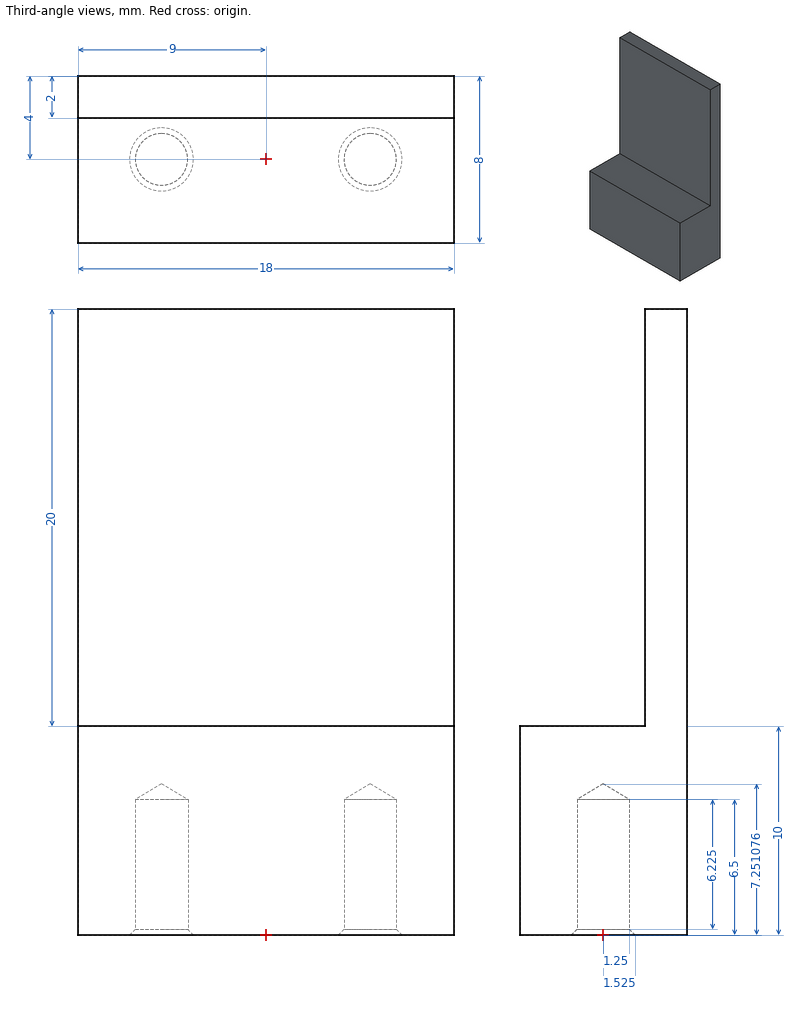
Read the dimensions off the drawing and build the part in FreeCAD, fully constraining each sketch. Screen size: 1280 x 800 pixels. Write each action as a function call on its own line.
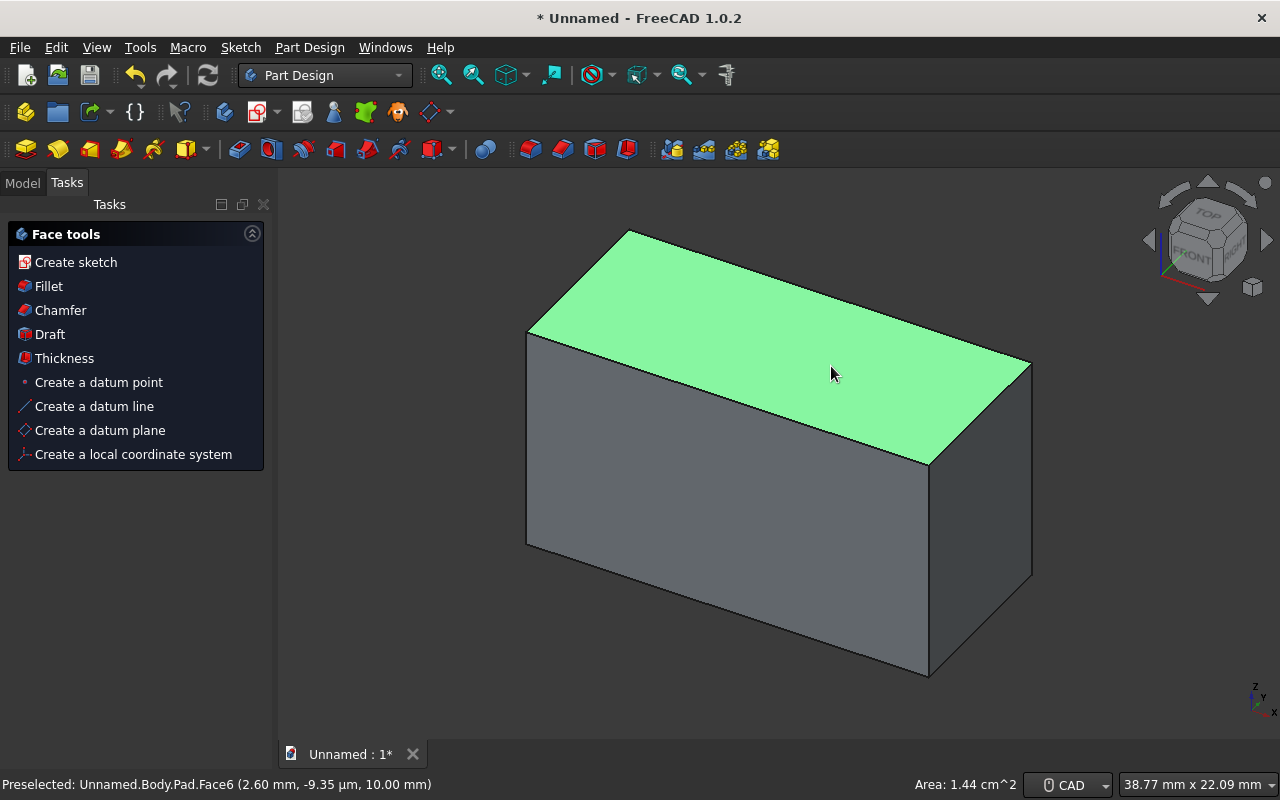
click(258, 112)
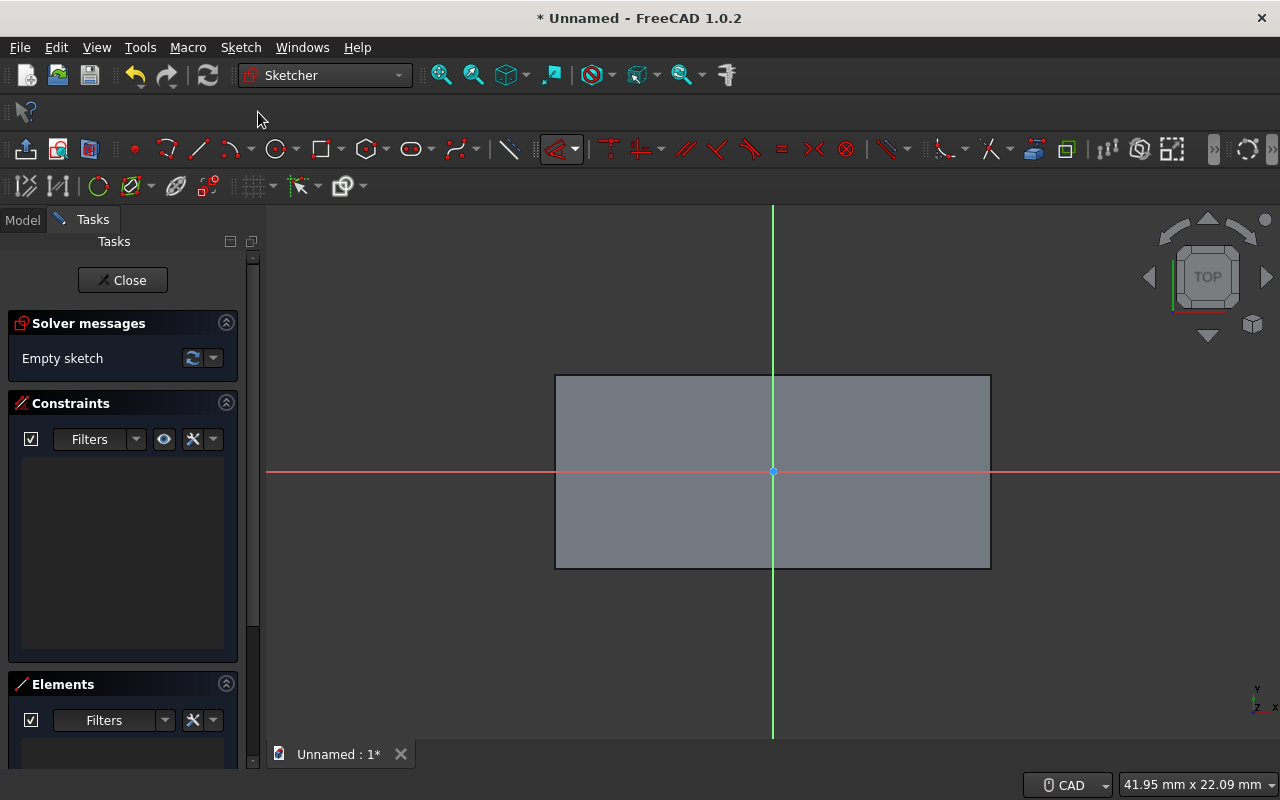
key(g)
key(r)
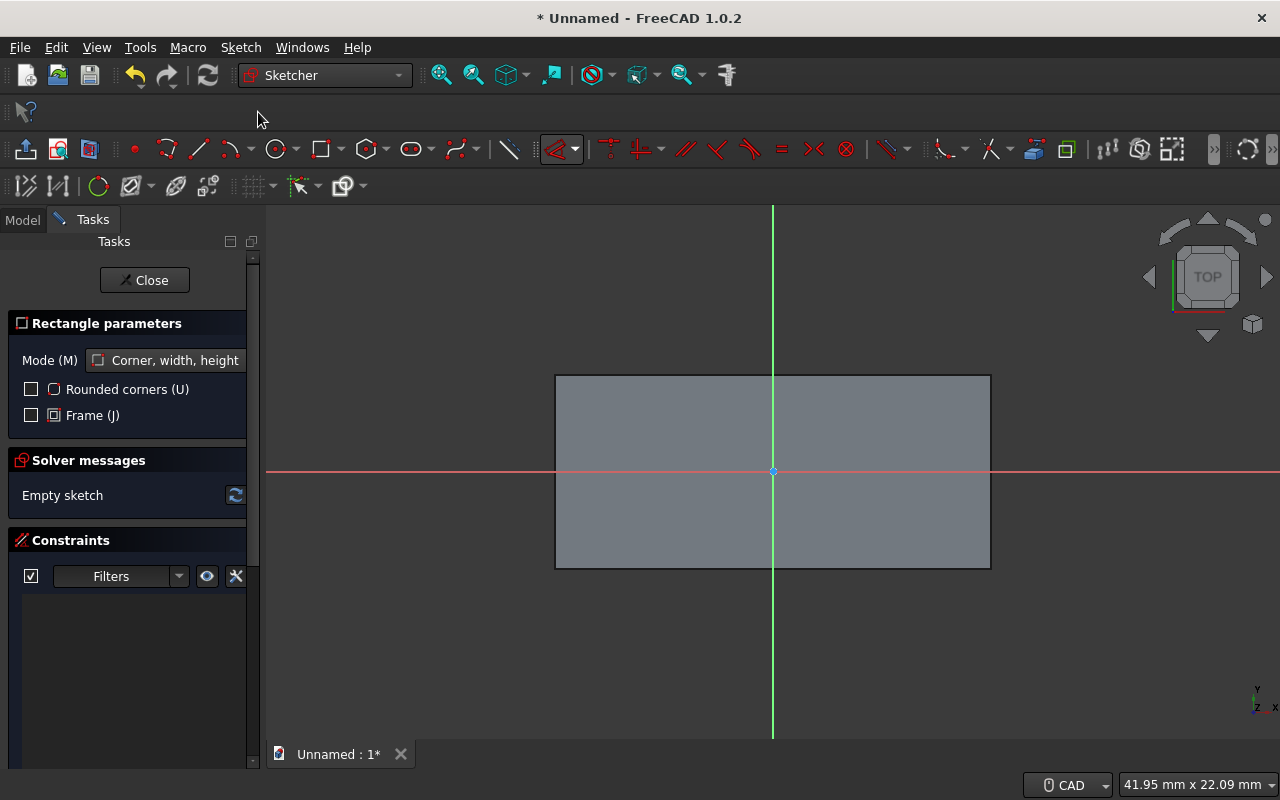
click(555, 375)
click(991, 424)
key(Escape)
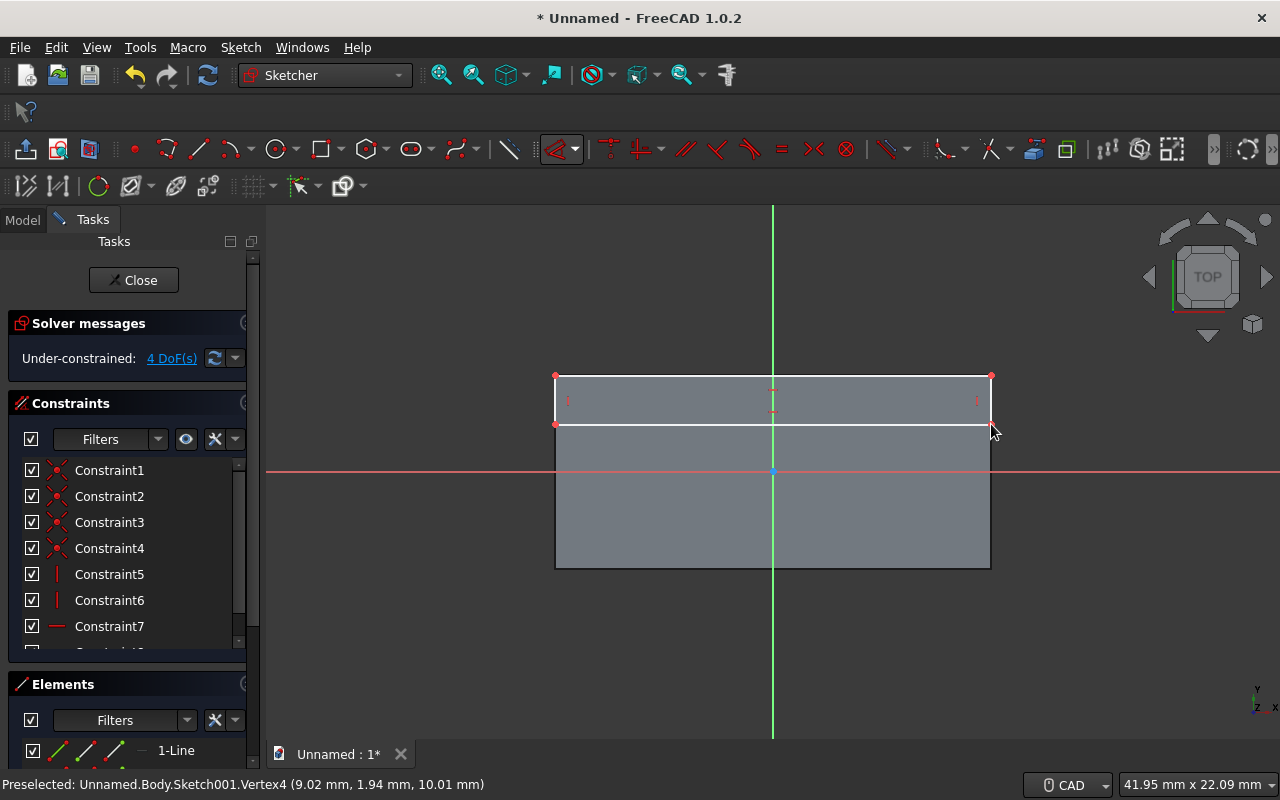
click(555, 391)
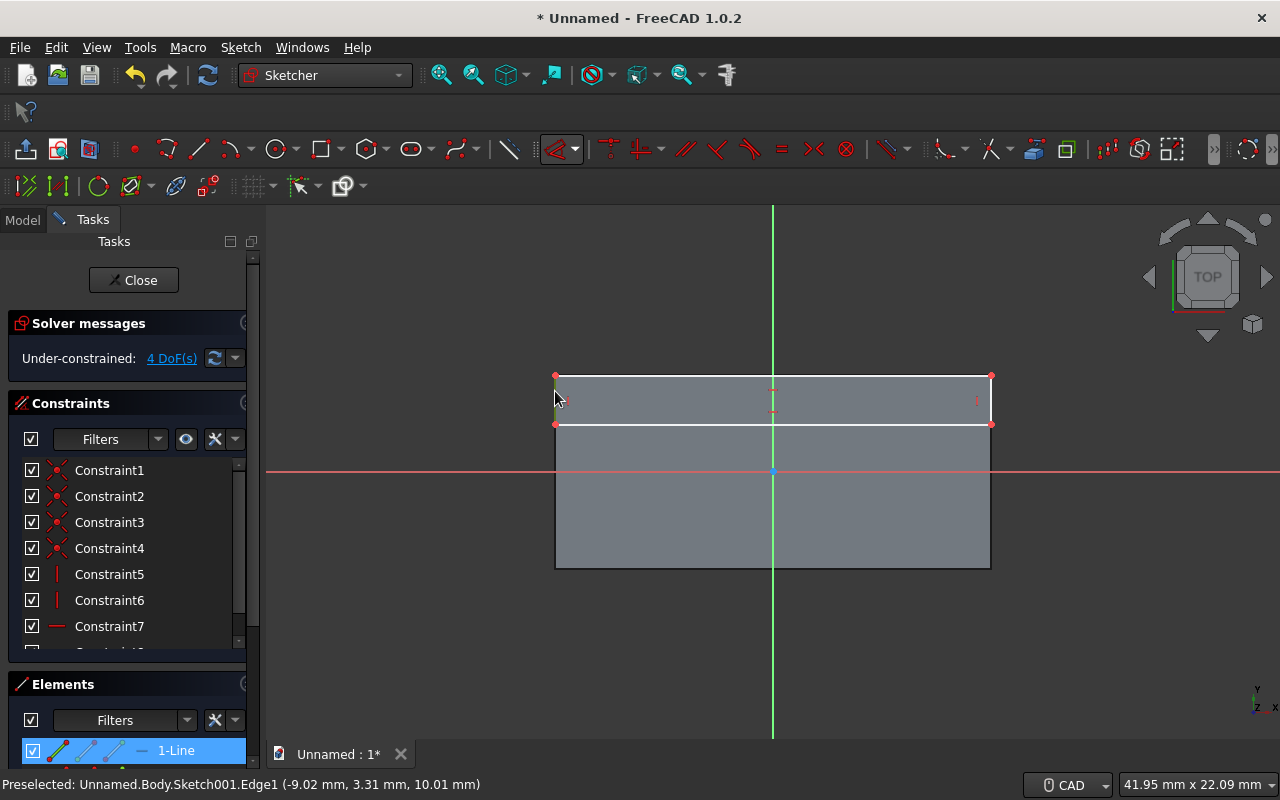
click(578, 150)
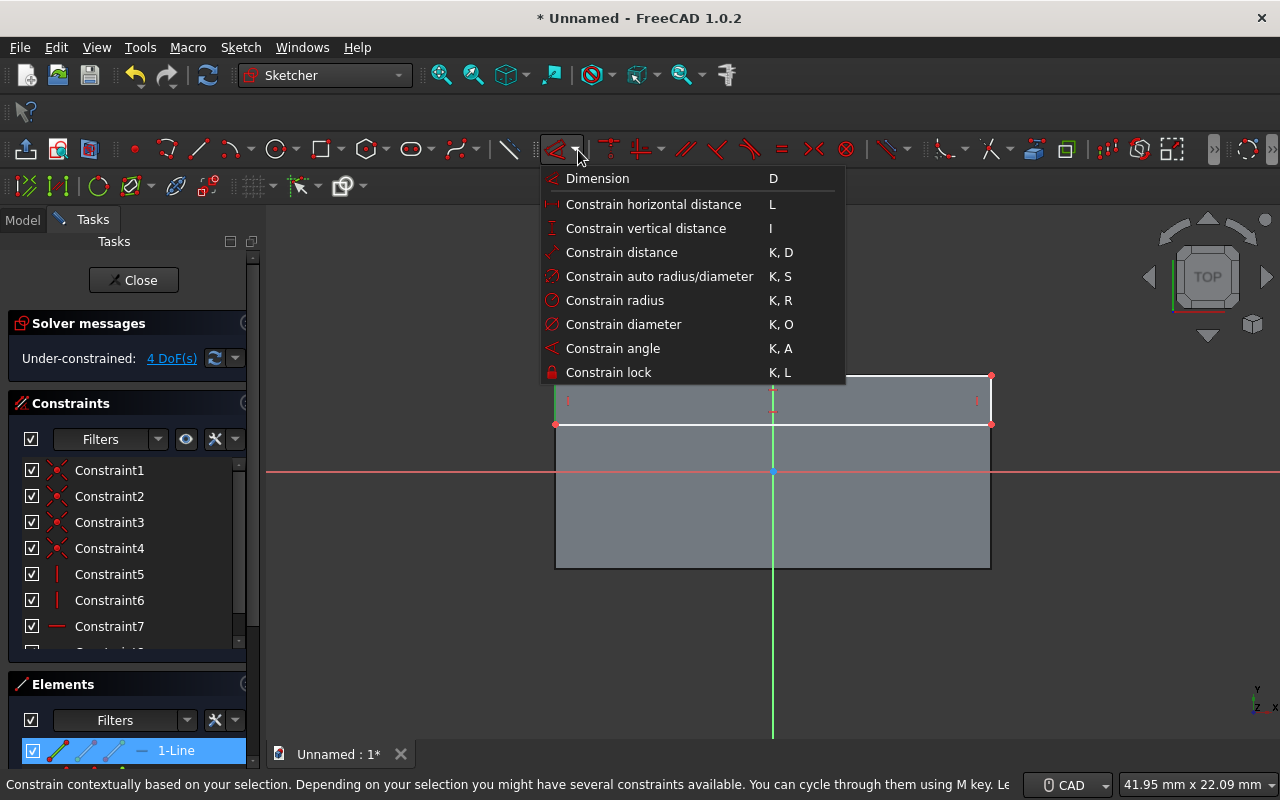
click(693, 228)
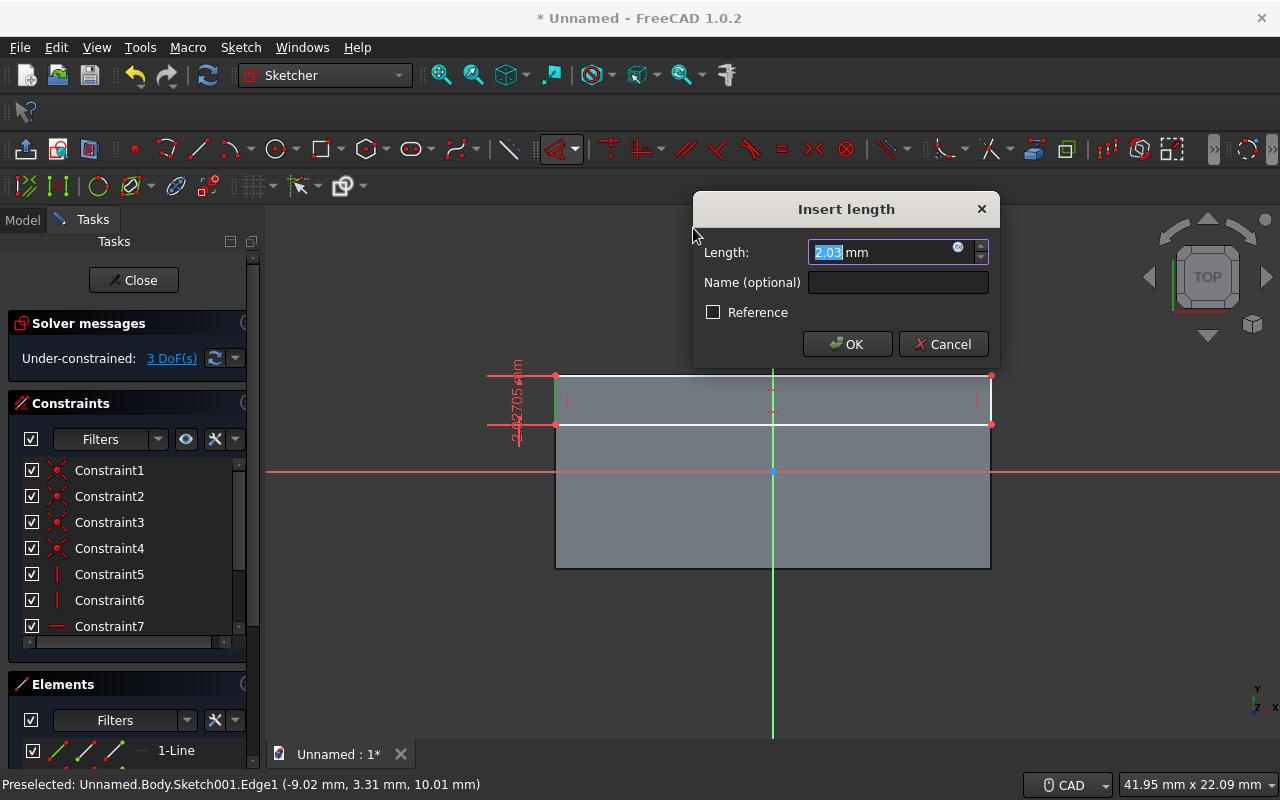
text(2)
key(Return)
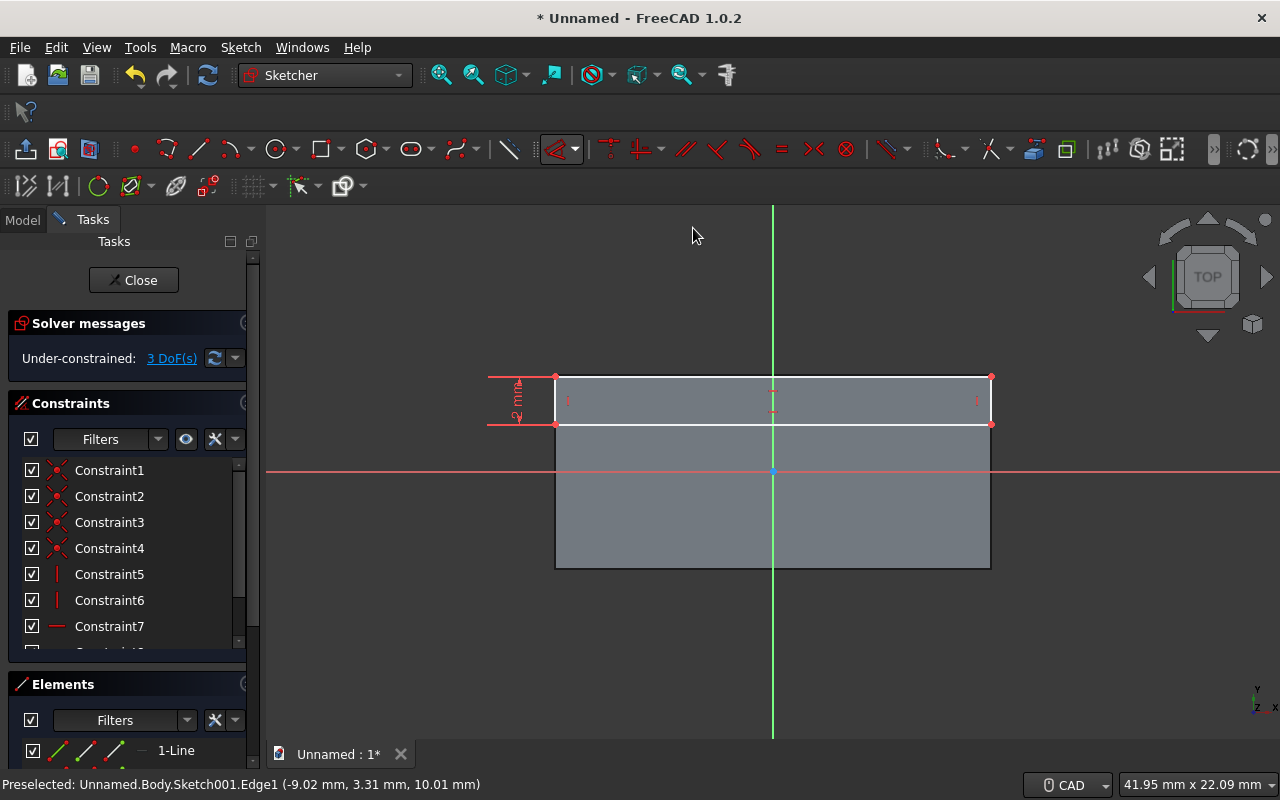
click(686, 425)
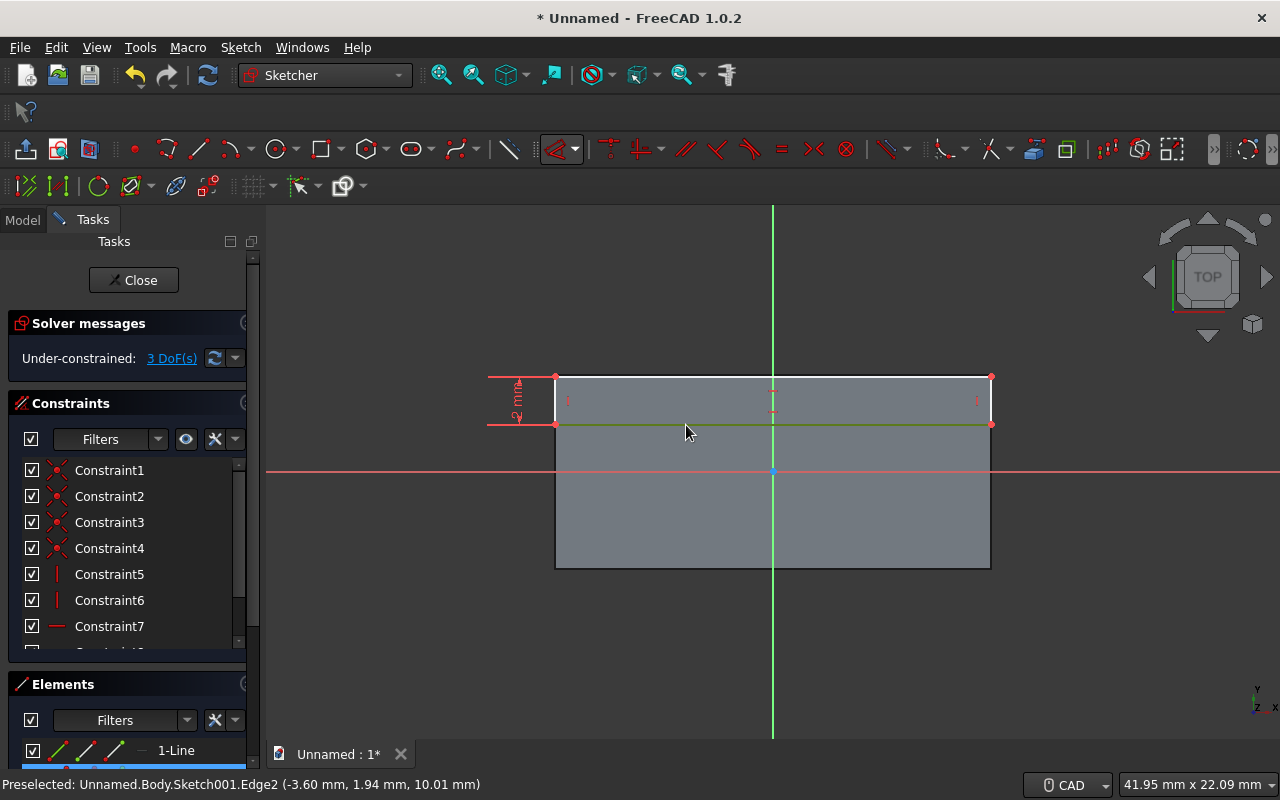
key(l)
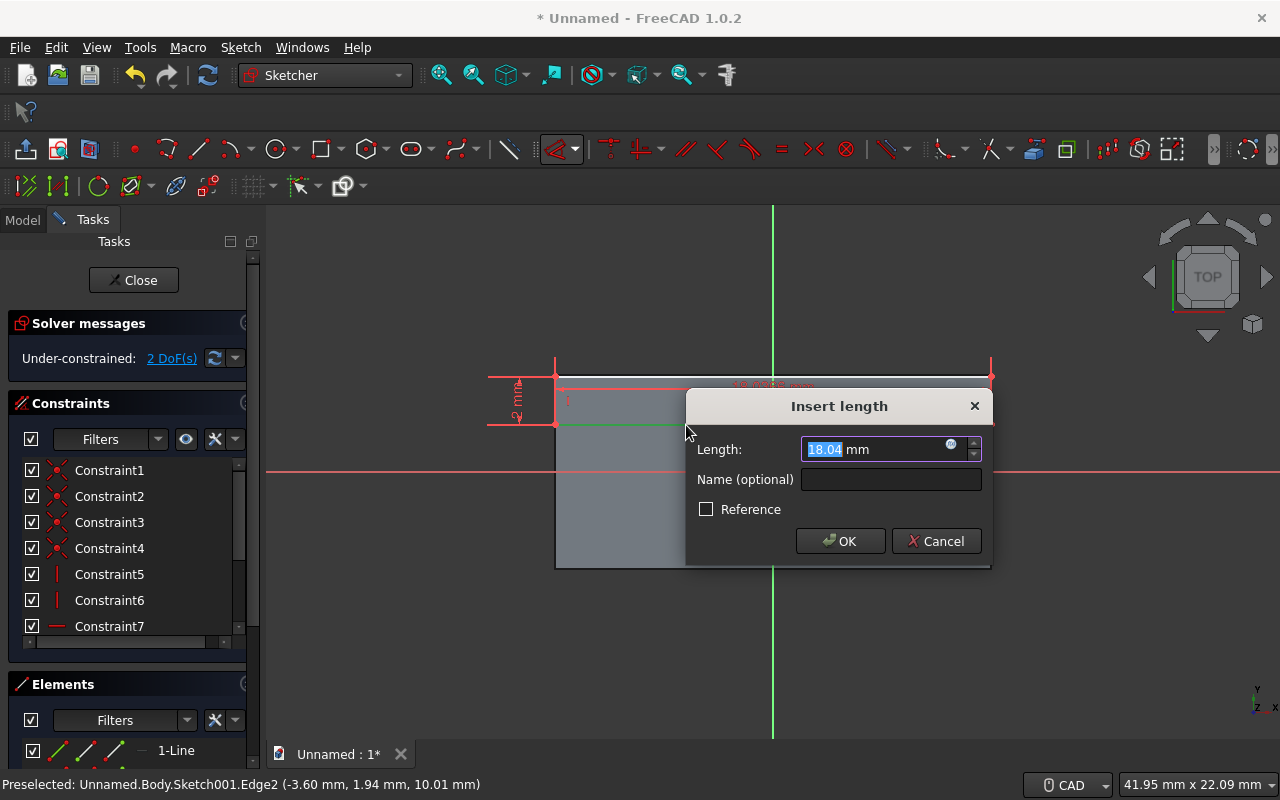
text(18)
key(Return)